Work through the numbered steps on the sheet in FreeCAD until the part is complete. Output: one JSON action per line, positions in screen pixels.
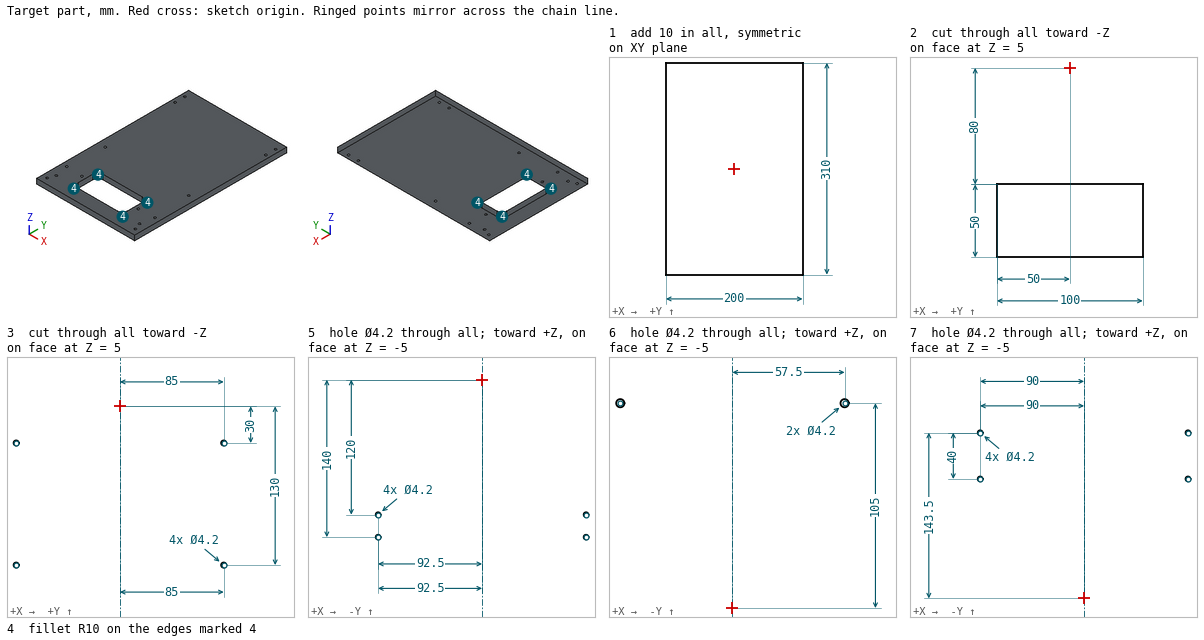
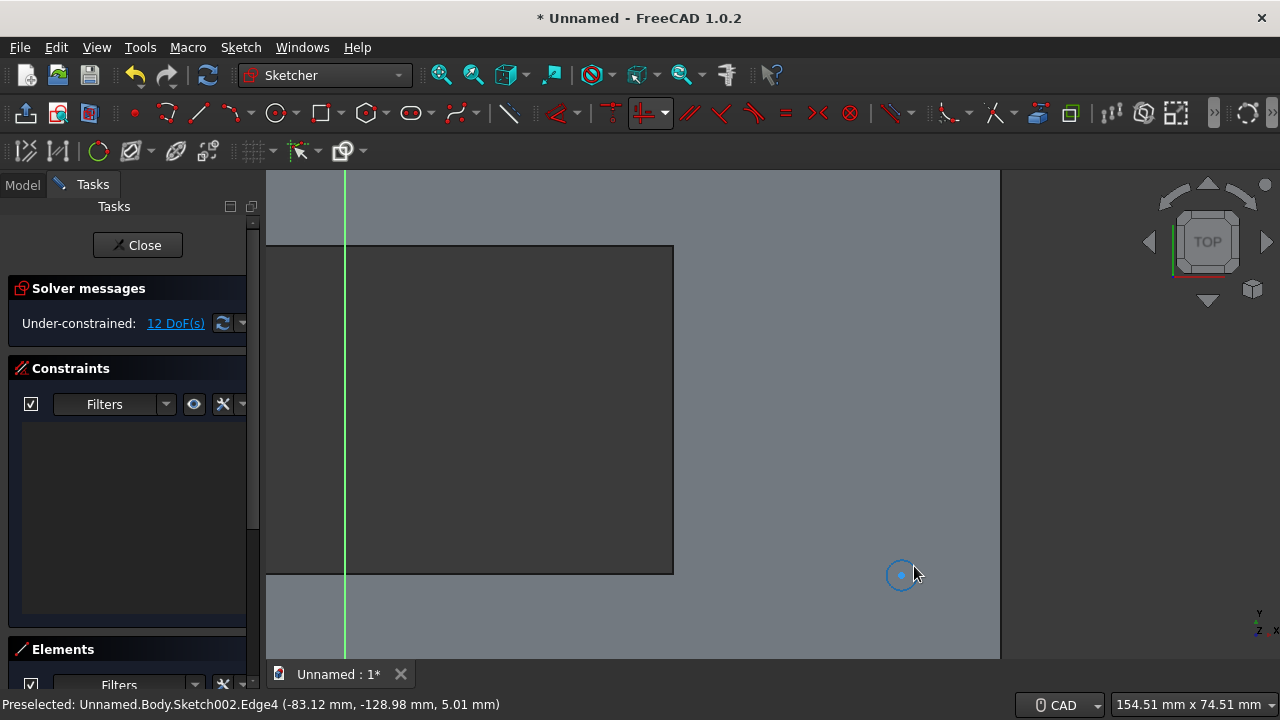
{"action": "left_click", "coordinate": [912, 565]}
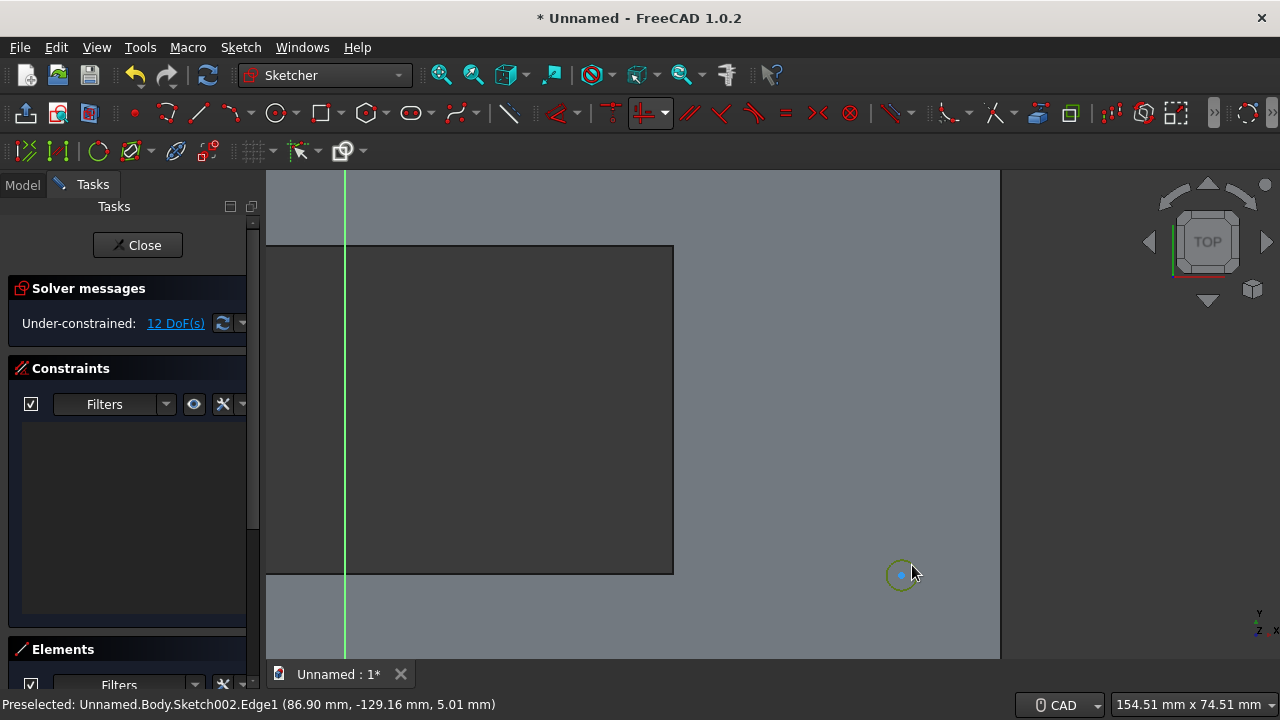
{"action": "scroll", "coordinate": [914, 566], "scroll_direction": "down", "scroll_amount": 5}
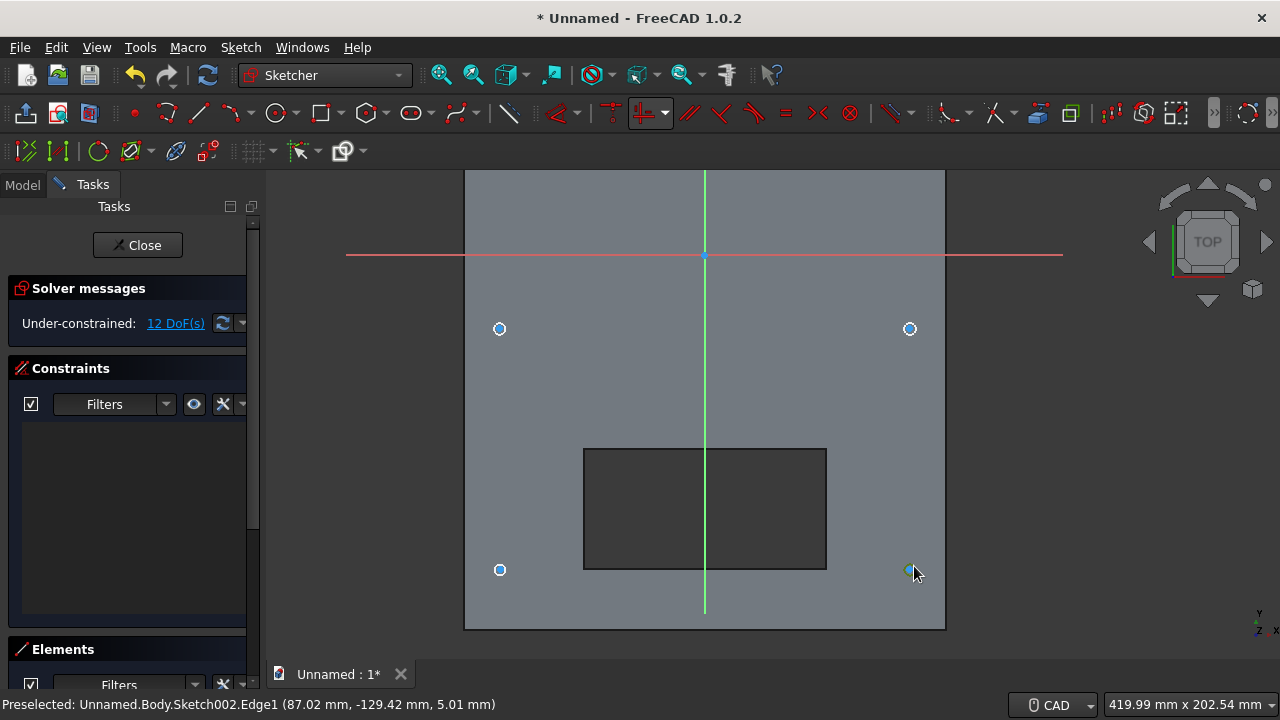
{"action": "scroll", "coordinate": [914, 325], "scroll_direction": "up", "scroll_amount": 5}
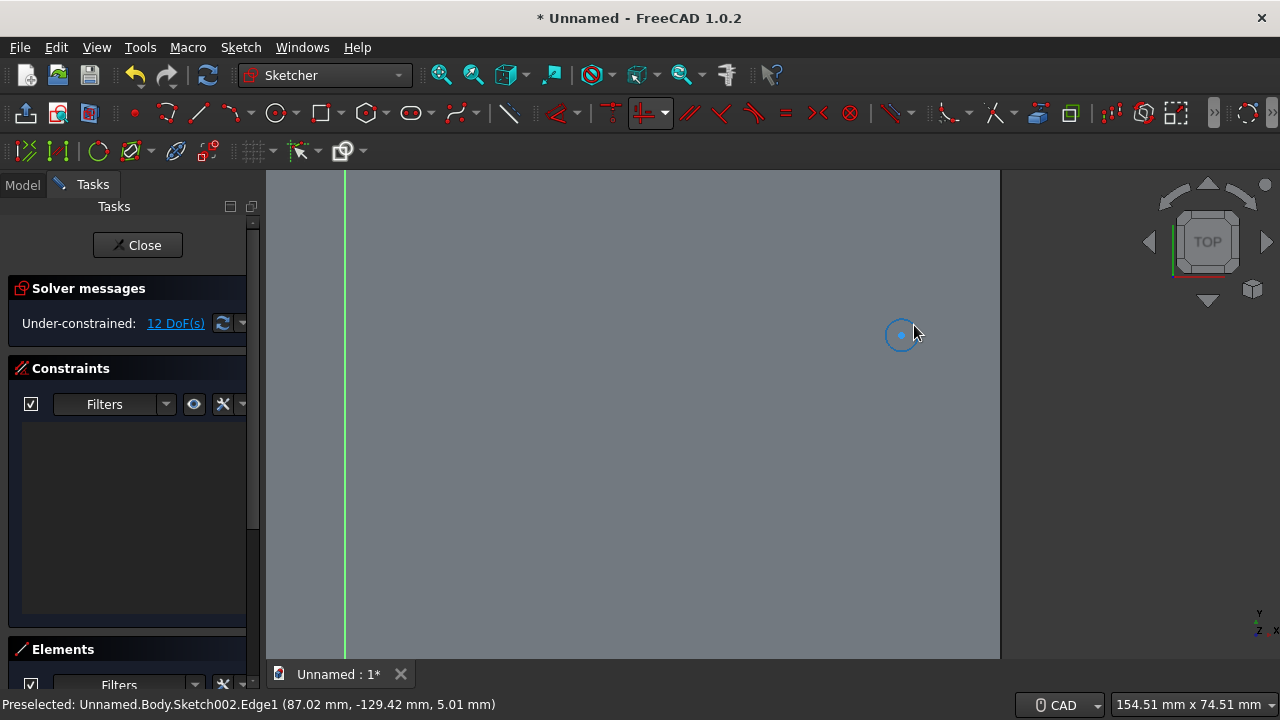
{"action": "left_click", "coordinate": [913, 324]}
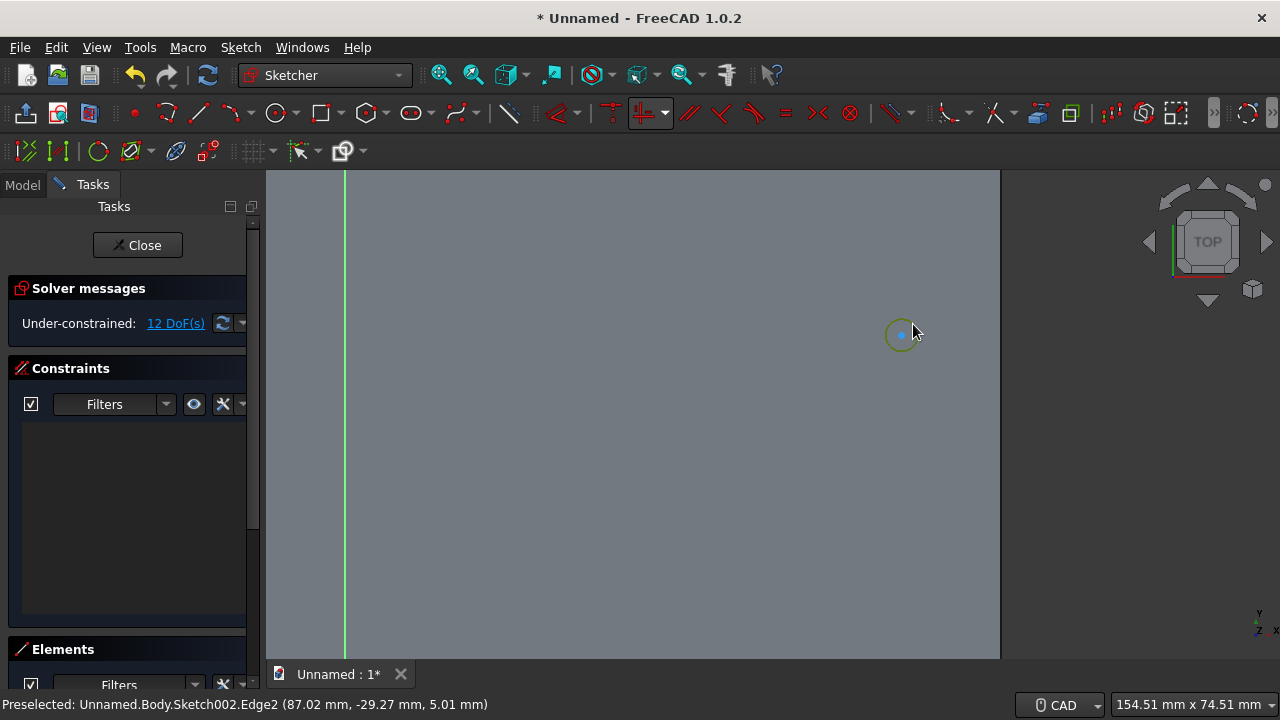
{"action": "scroll", "coordinate": [914, 325], "scroll_direction": "down", "scroll_amount": 5}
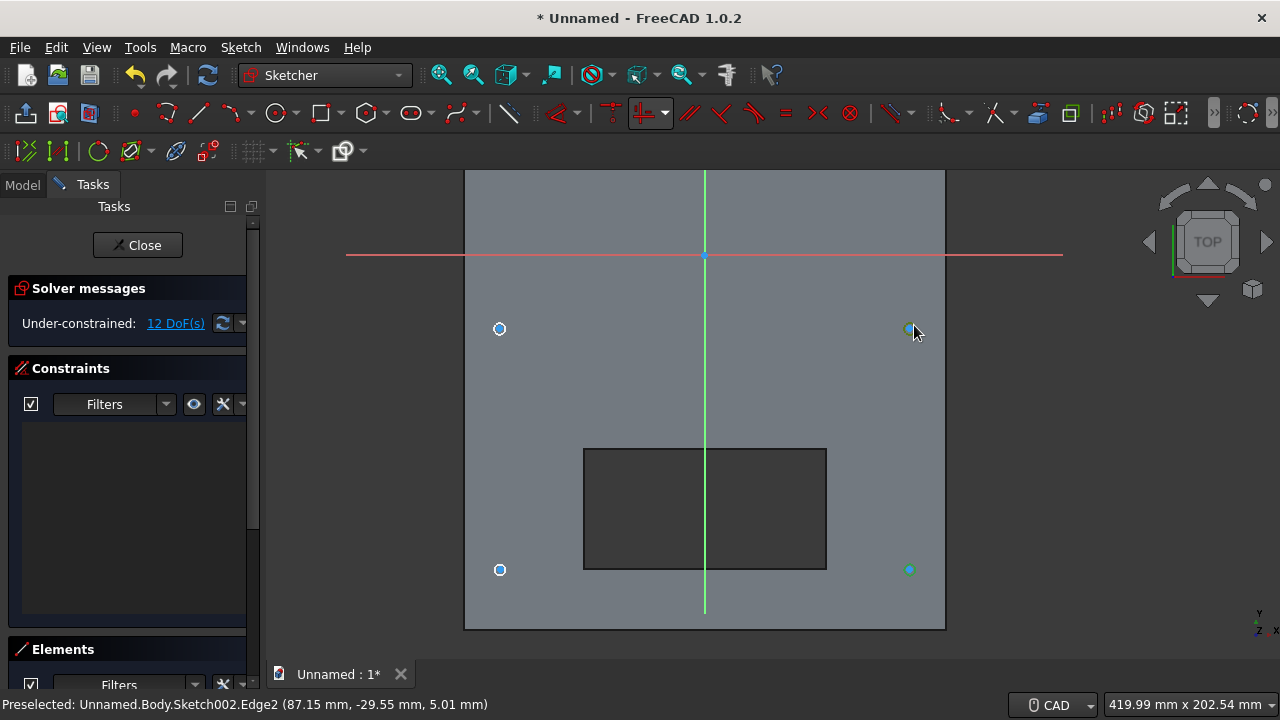
{"action": "scroll", "coordinate": [504, 325], "scroll_direction": "up", "scroll_amount": 5}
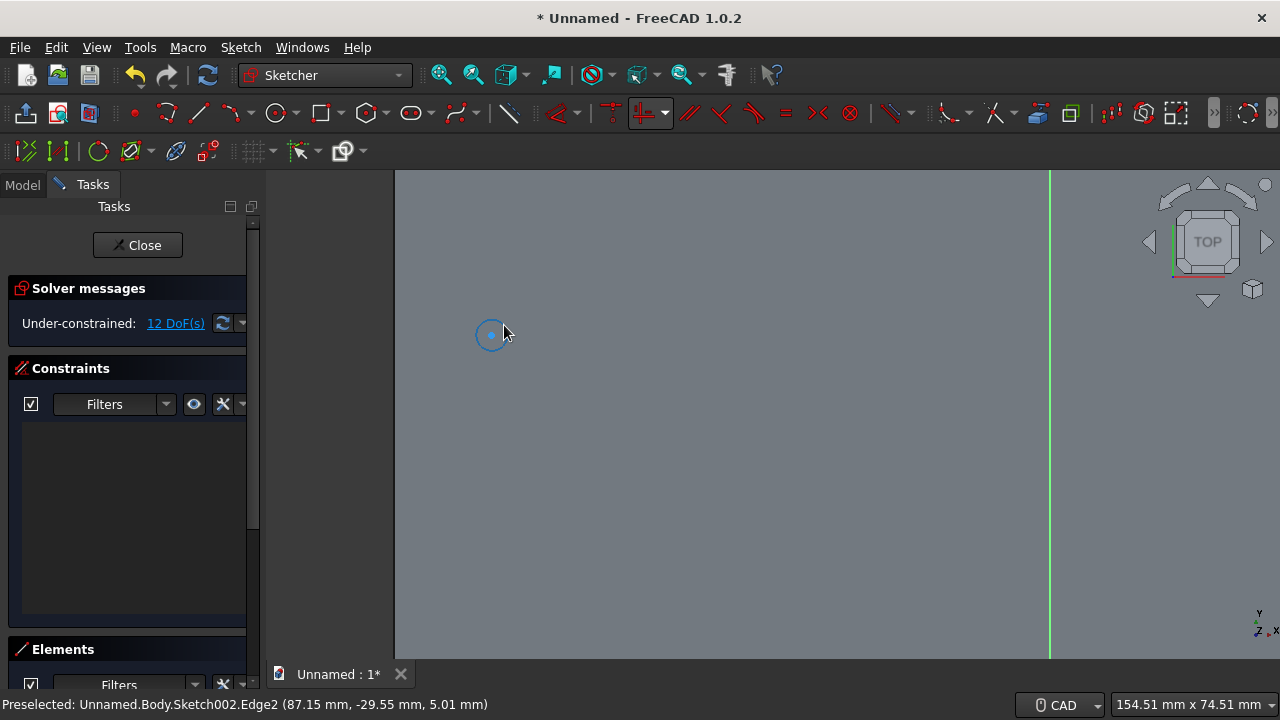
{"action": "left_click", "coordinate": [503, 324]}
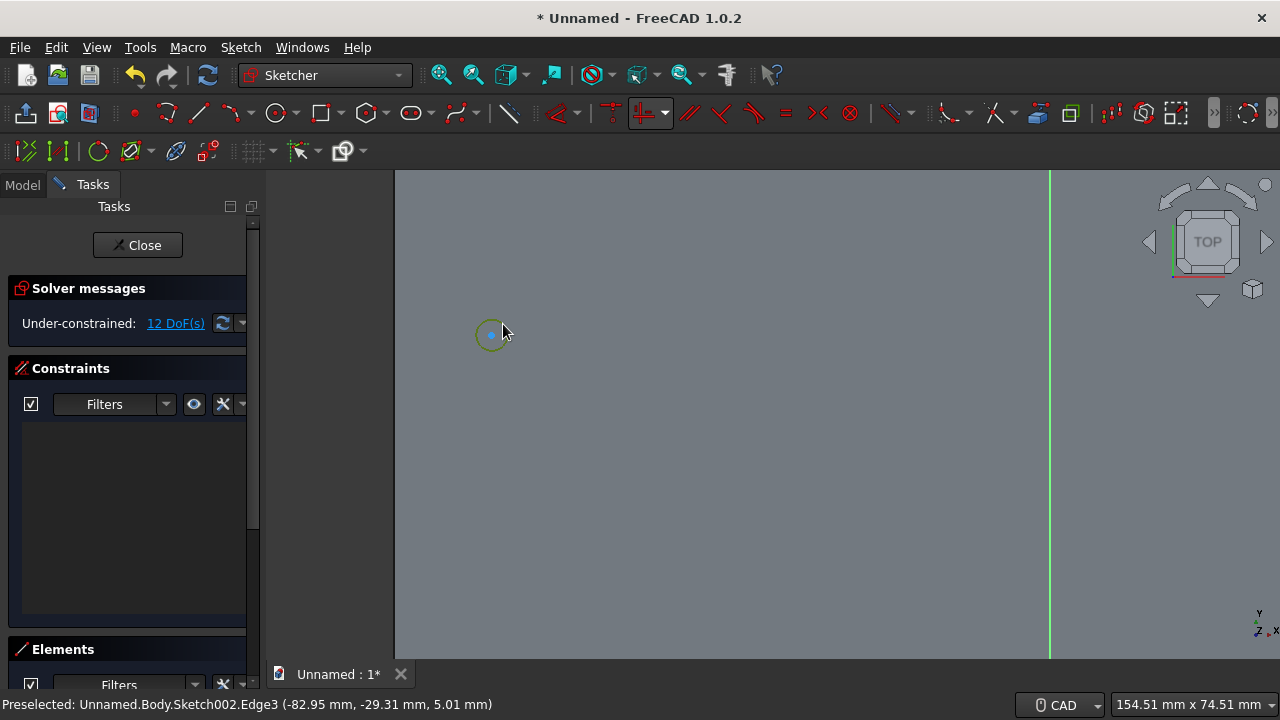
{"action": "scroll", "coordinate": [503, 325], "scroll_direction": "down", "scroll_amount": 5}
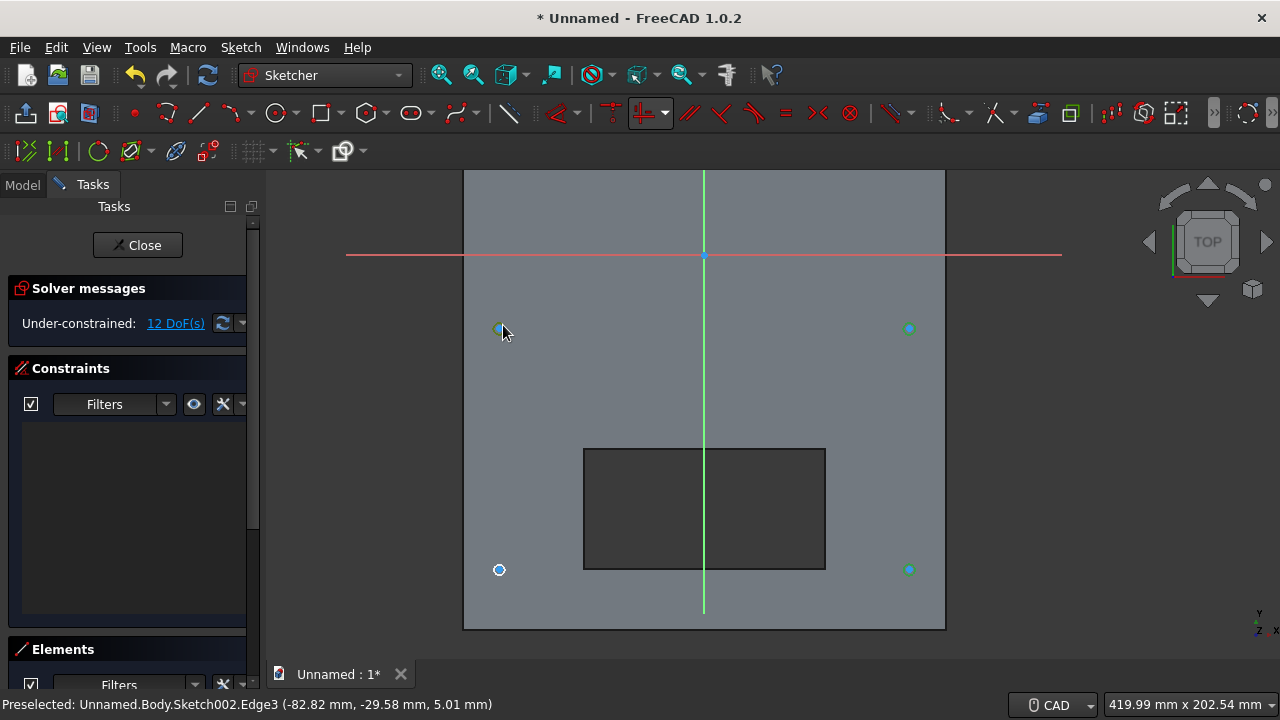
{"action": "scroll", "coordinate": [503, 566], "scroll_direction": "up", "scroll_amount": 5}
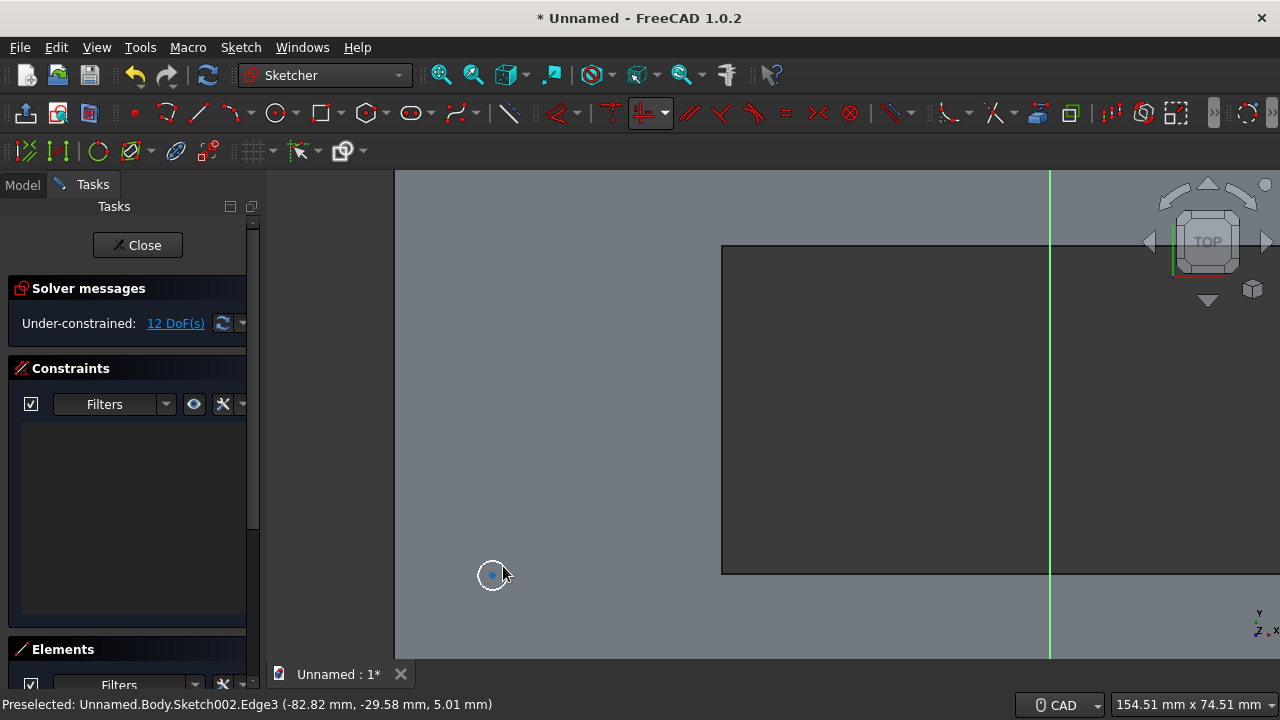
{"action": "left_click", "coordinate": [503, 565]}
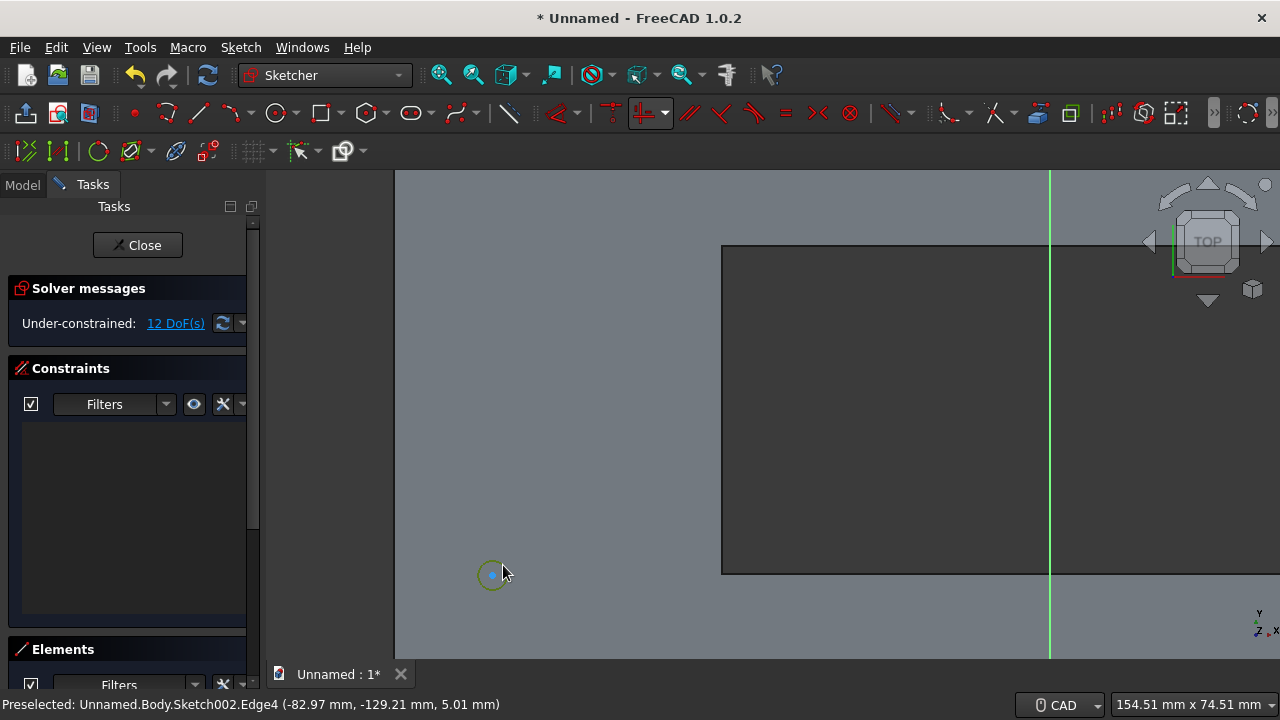
{"action": "left_click", "coordinate": [786, 114]}